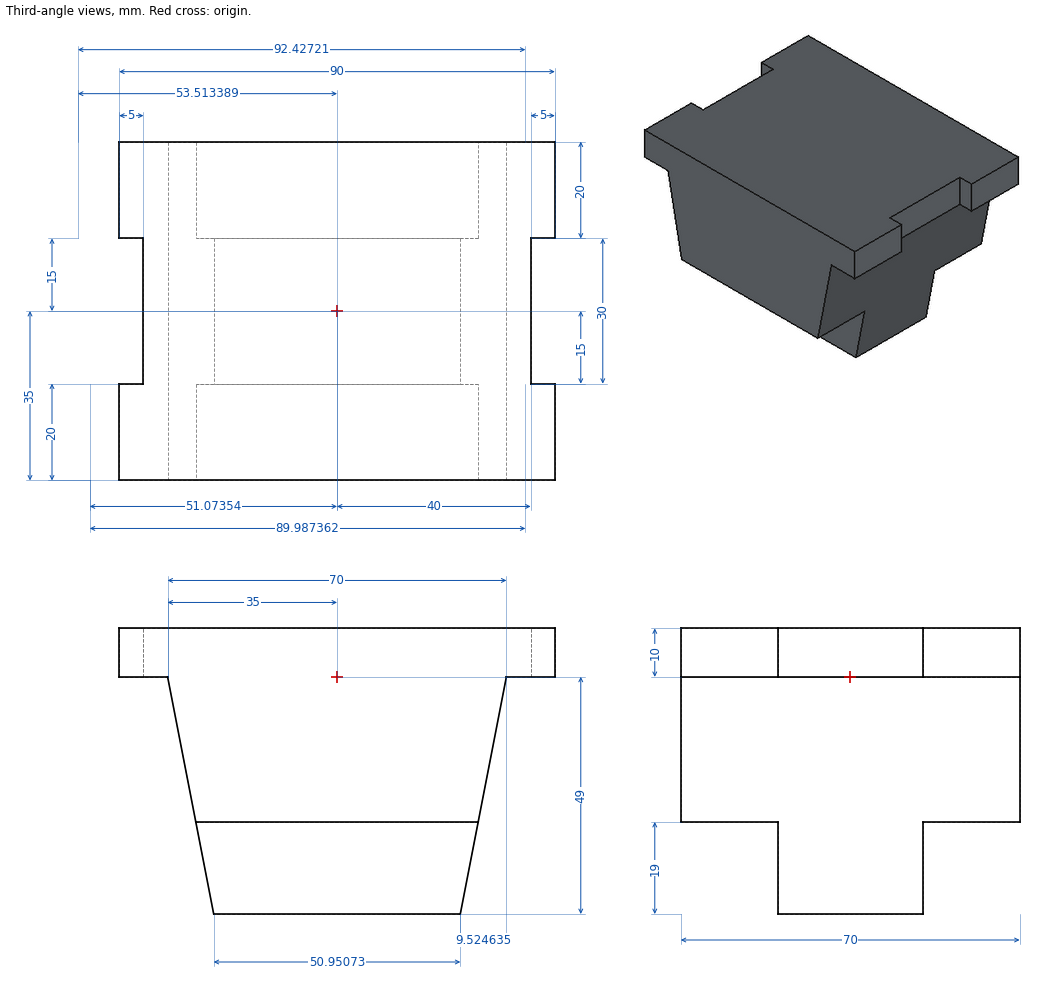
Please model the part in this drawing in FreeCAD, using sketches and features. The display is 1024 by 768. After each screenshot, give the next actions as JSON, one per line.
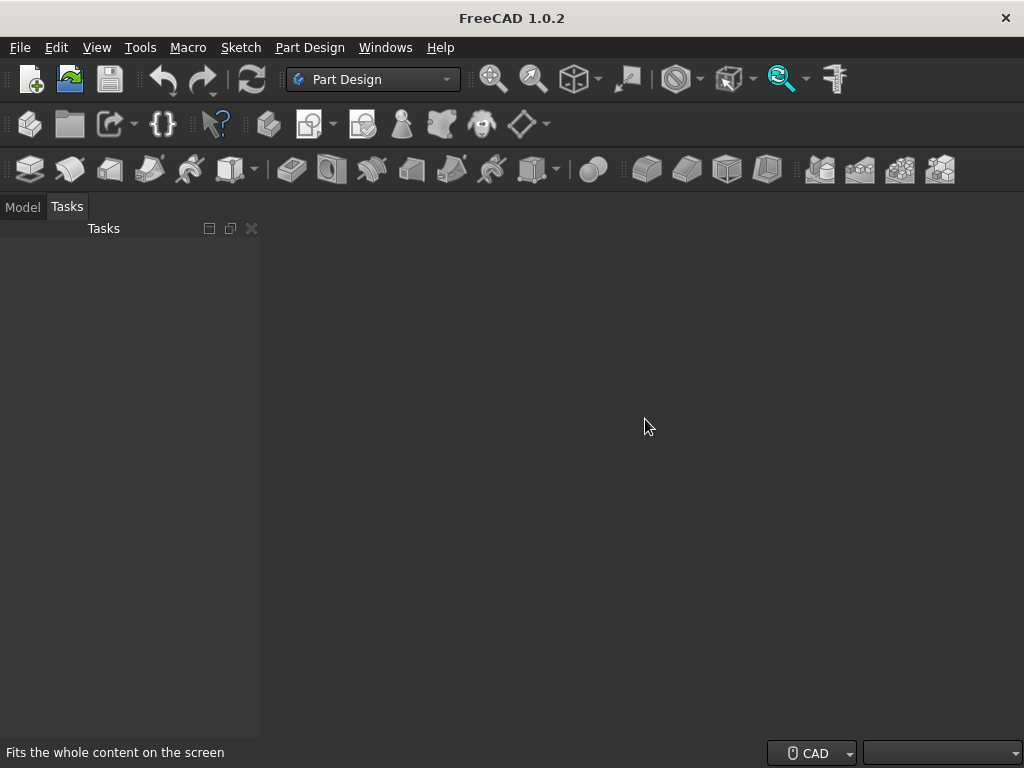
{"action": "key", "text": "ctrl+n"}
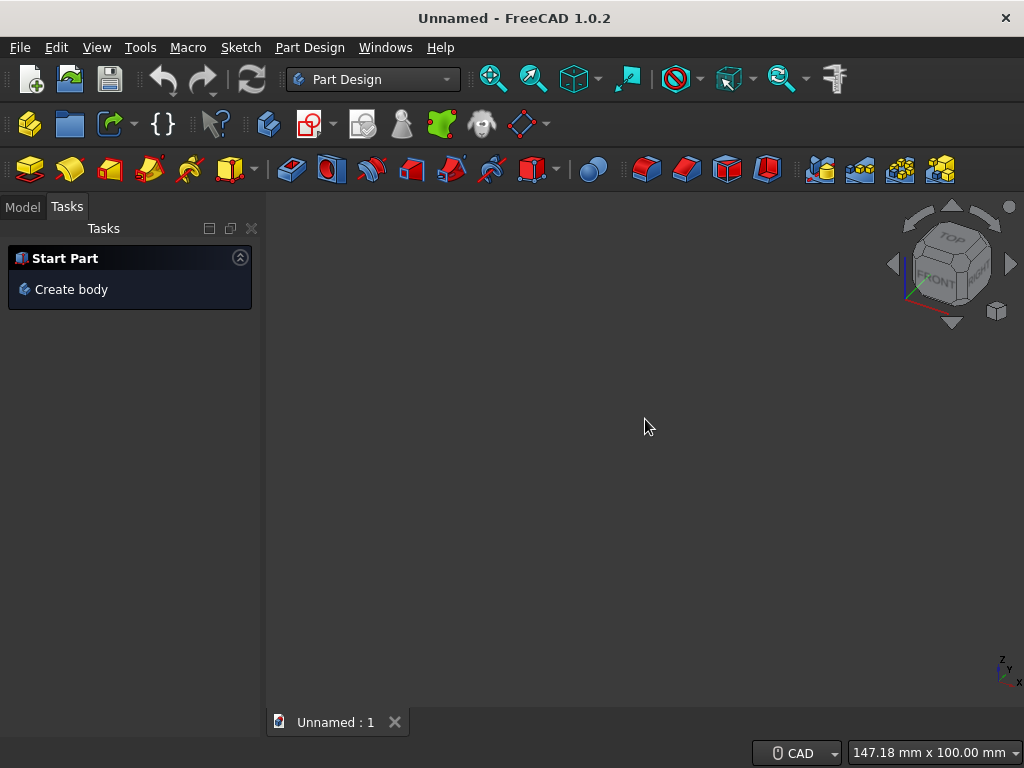
{"action": "left_click", "coordinate": [310, 124]}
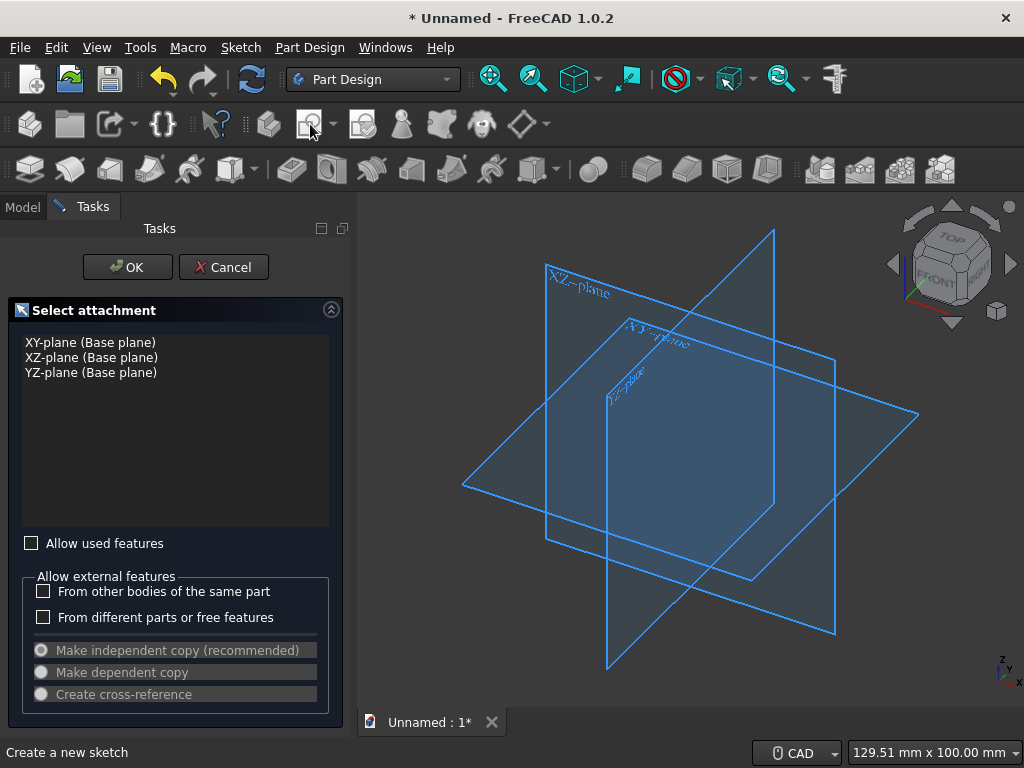
{"action": "left_click", "coordinate": [82, 342]}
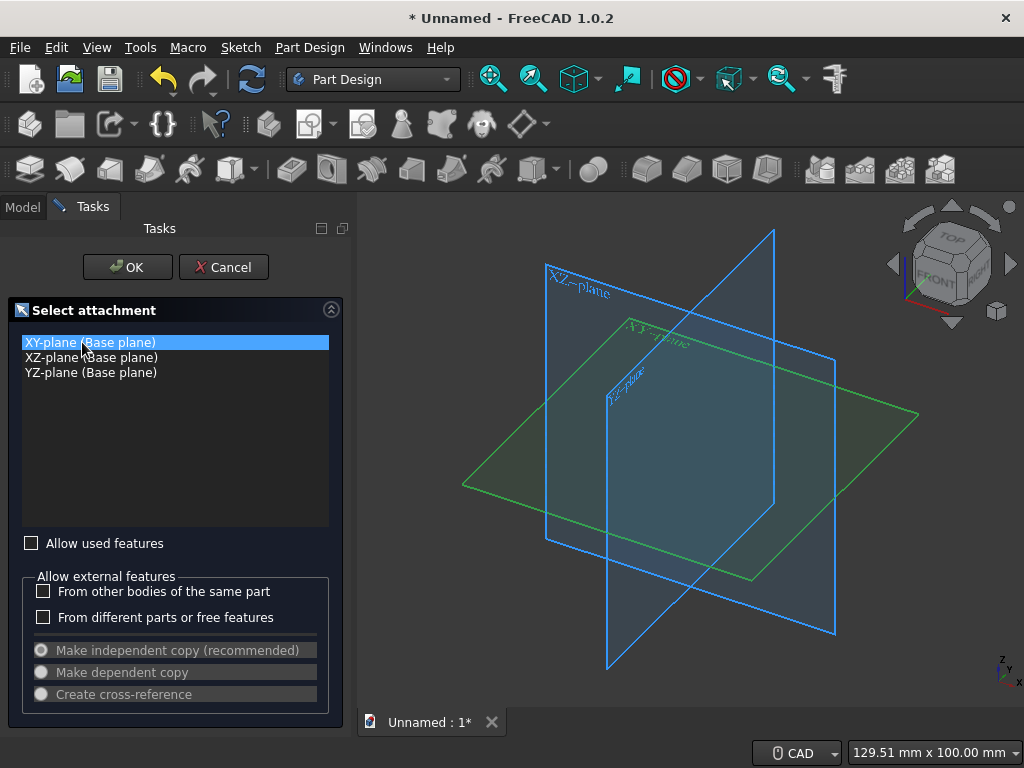
{"action": "left_click", "coordinate": [128, 267]}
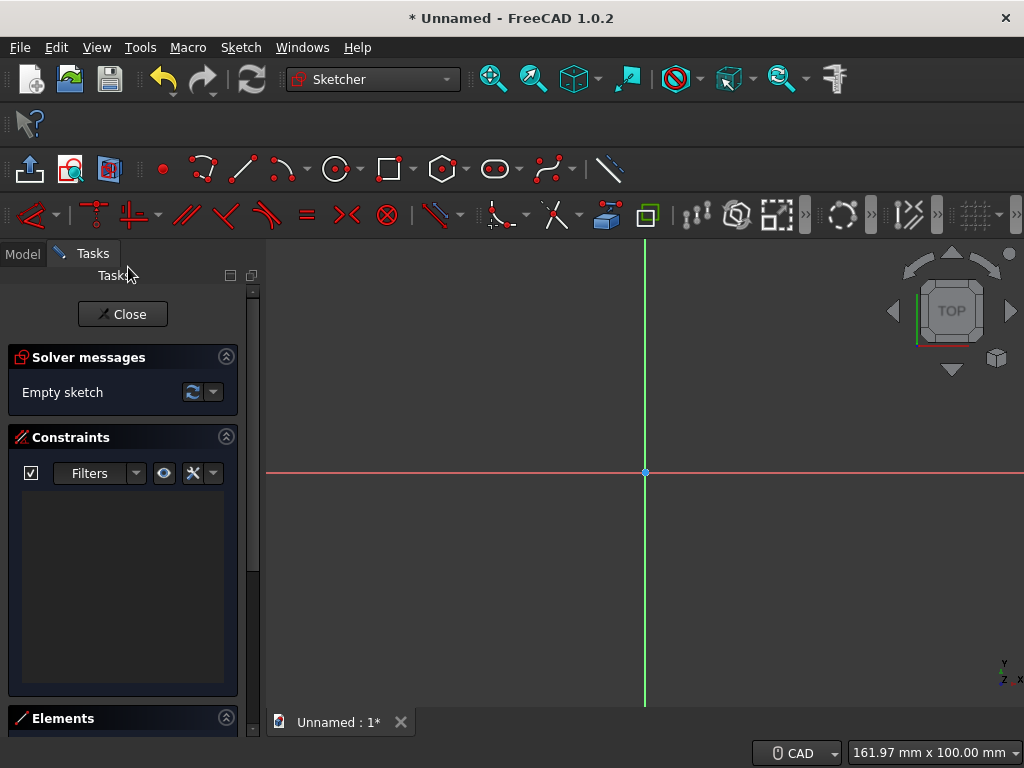
{"action": "scroll", "coordinate": [294, 473], "scroll_direction": "down", "scroll_amount": 1}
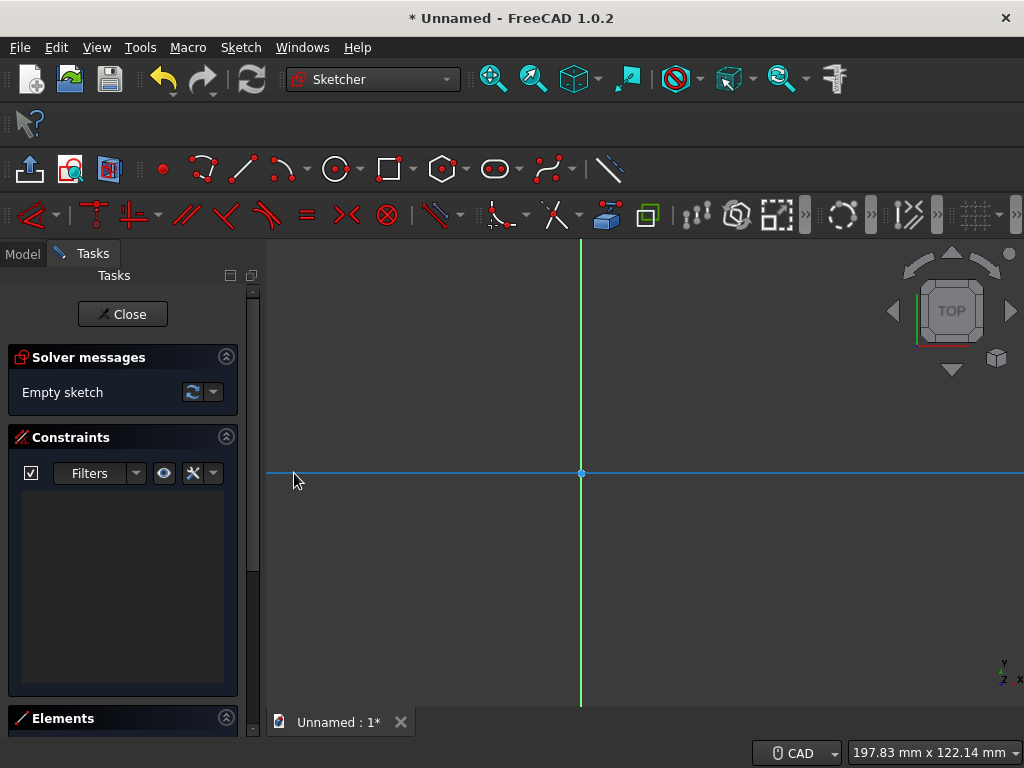
{"action": "key", "text": "g m"}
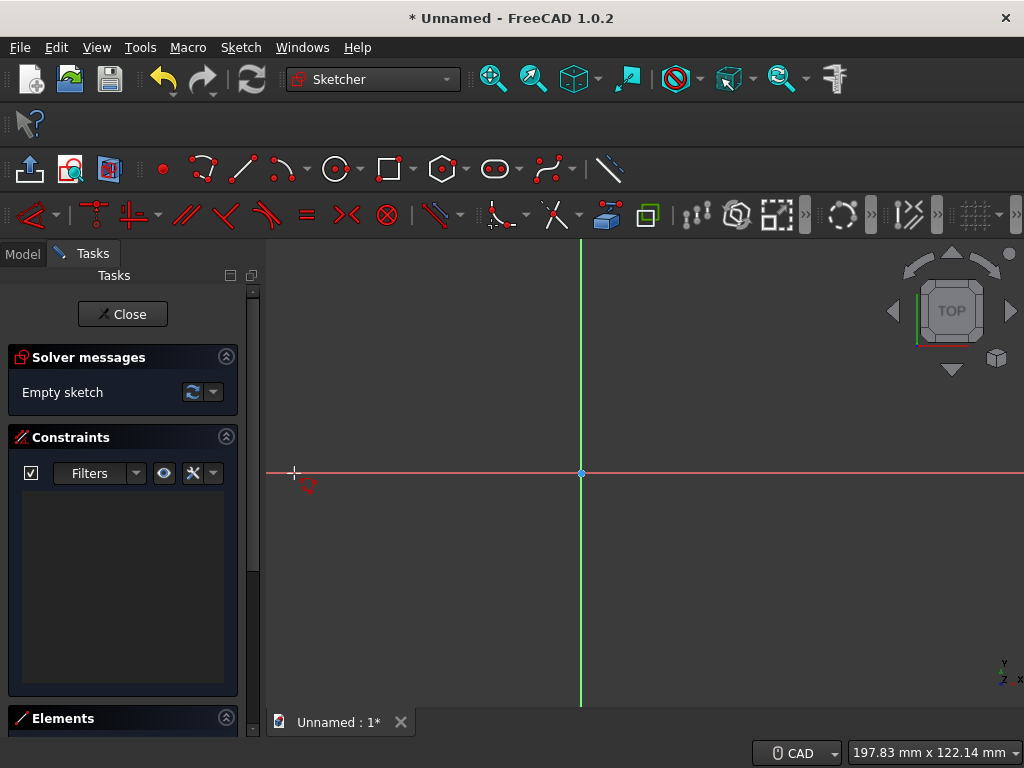
{"action": "left_click", "coordinate": [735, 531]}
{"action": "left_click", "coordinate": [735, 416]}
{"action": "left_click", "coordinate": [754, 416]}
{"action": "left_click", "coordinate": [754, 339]}
{"action": "left_click", "coordinate": [409, 339]}
{"action": "left_click", "coordinate": [409, 416]}
{"action": "left_click", "coordinate": [428, 416]}
{"action": "left_click", "coordinate": [428, 531]}
{"action": "left_click", "coordinate": [409, 531]}
{"action": "left_click", "coordinate": [409, 607]}
{"action": "left_click", "coordinate": [754, 607]}
{"action": "left_click", "coordinate": [754, 531]}
{"action": "left_click", "coordinate": [735, 532]}
{"action": "key", "text": "Escape"}
{"action": "key", "text": "Escape"}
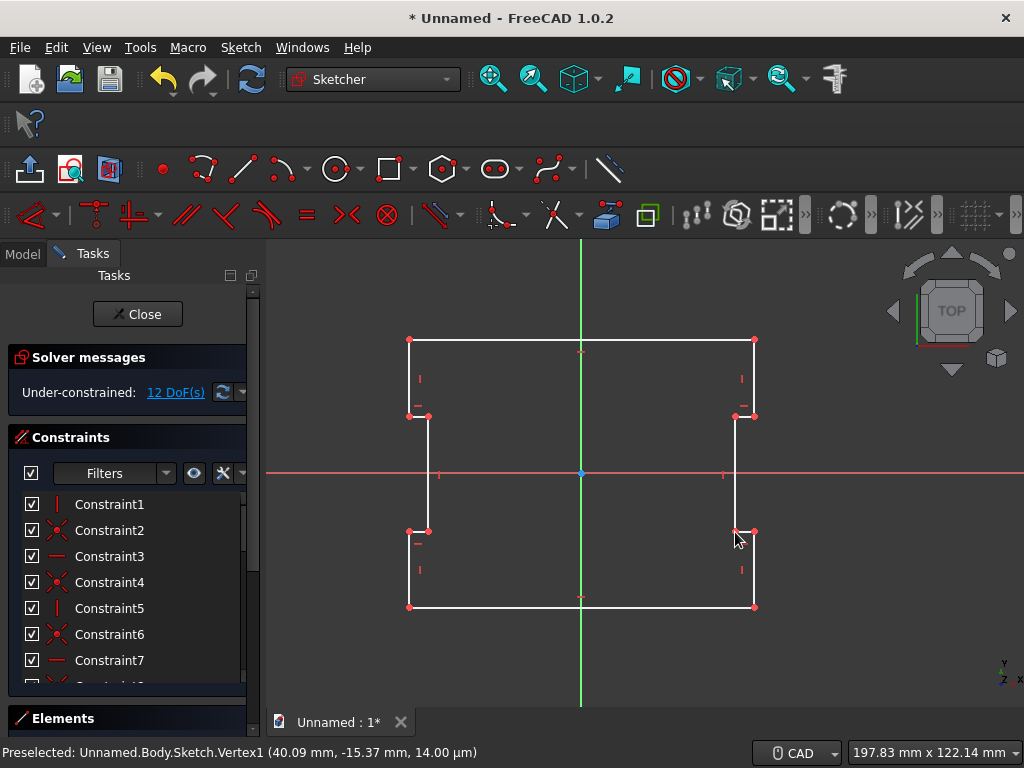
{"action": "key", "text": "d"}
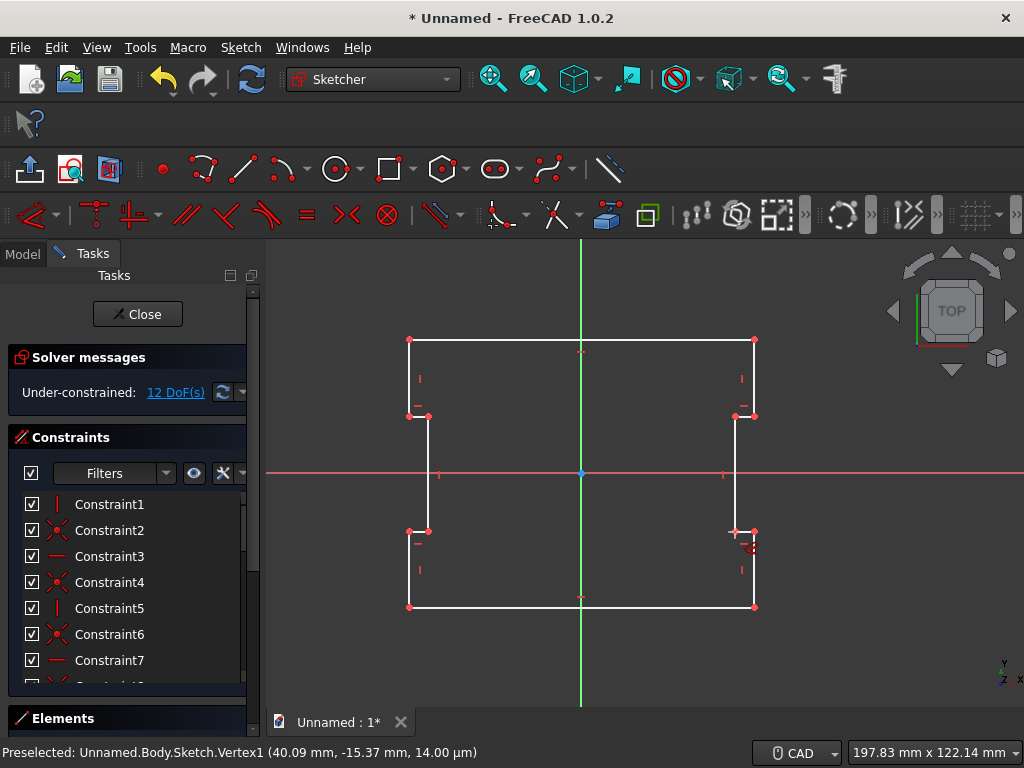
{"action": "scroll", "coordinate": [745, 417], "scroll_direction": "up", "scroll_amount": 4}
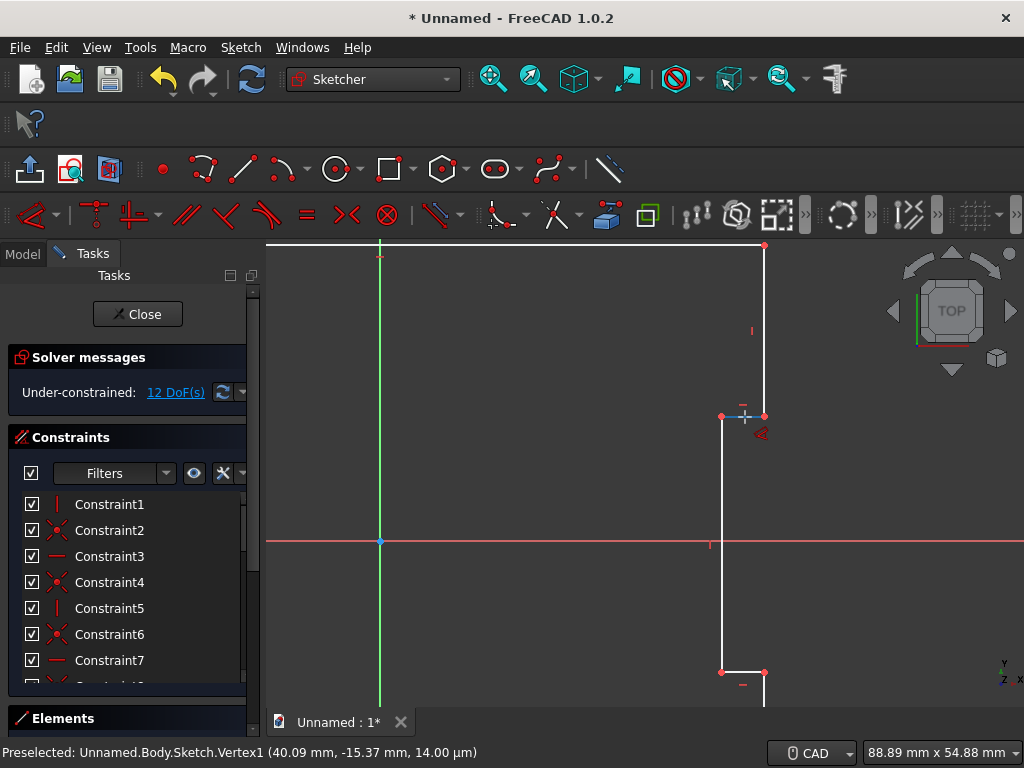
{"action": "left_click", "coordinate": [743, 417]}
{"action": "left_click", "coordinate": [743, 383]}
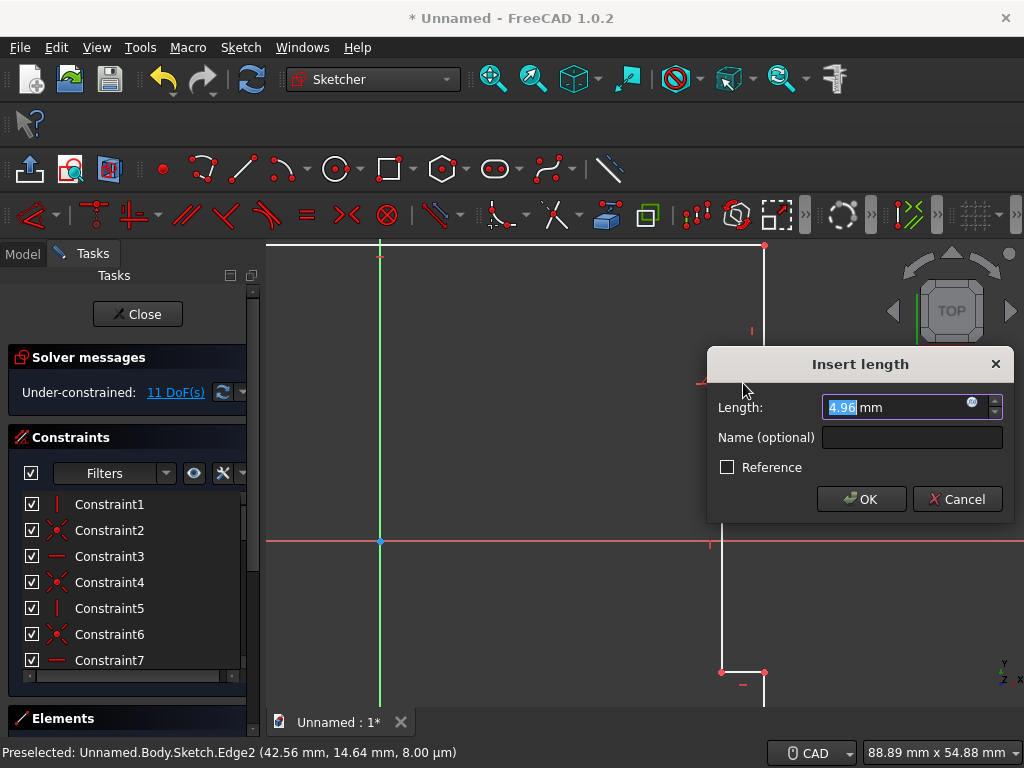
{"action": "type", "text": "5"}
{"action": "key", "text": "Return"}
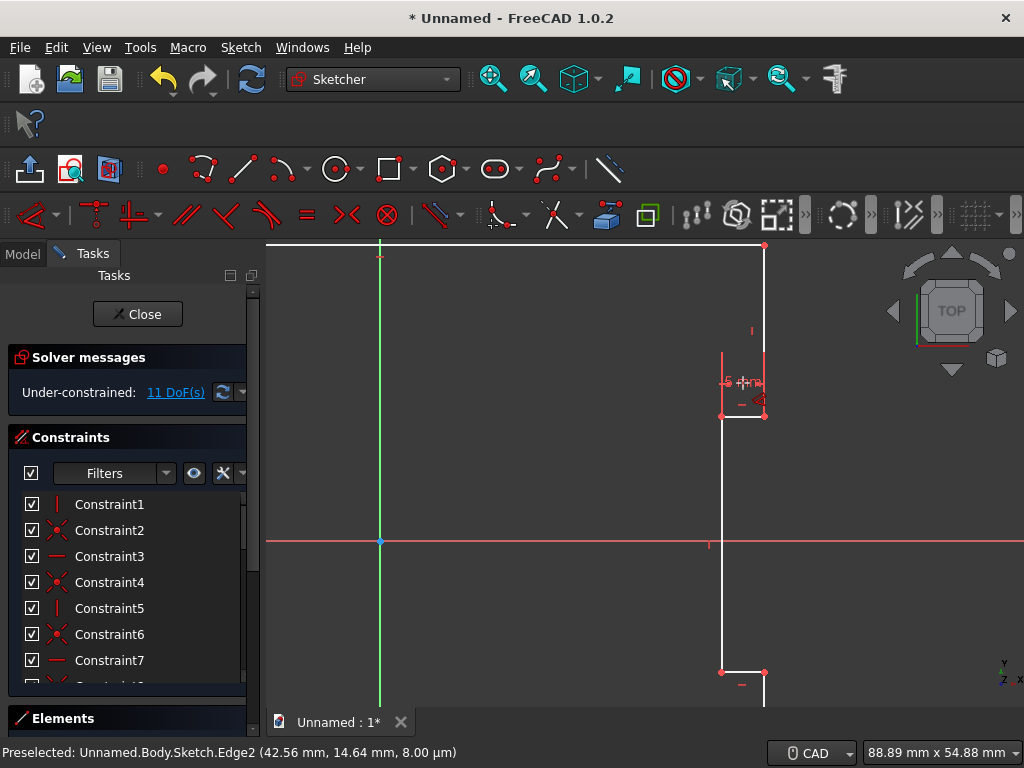
{"action": "scroll", "coordinate": [737, 417], "scroll_direction": "down", "scroll_amount": 4}